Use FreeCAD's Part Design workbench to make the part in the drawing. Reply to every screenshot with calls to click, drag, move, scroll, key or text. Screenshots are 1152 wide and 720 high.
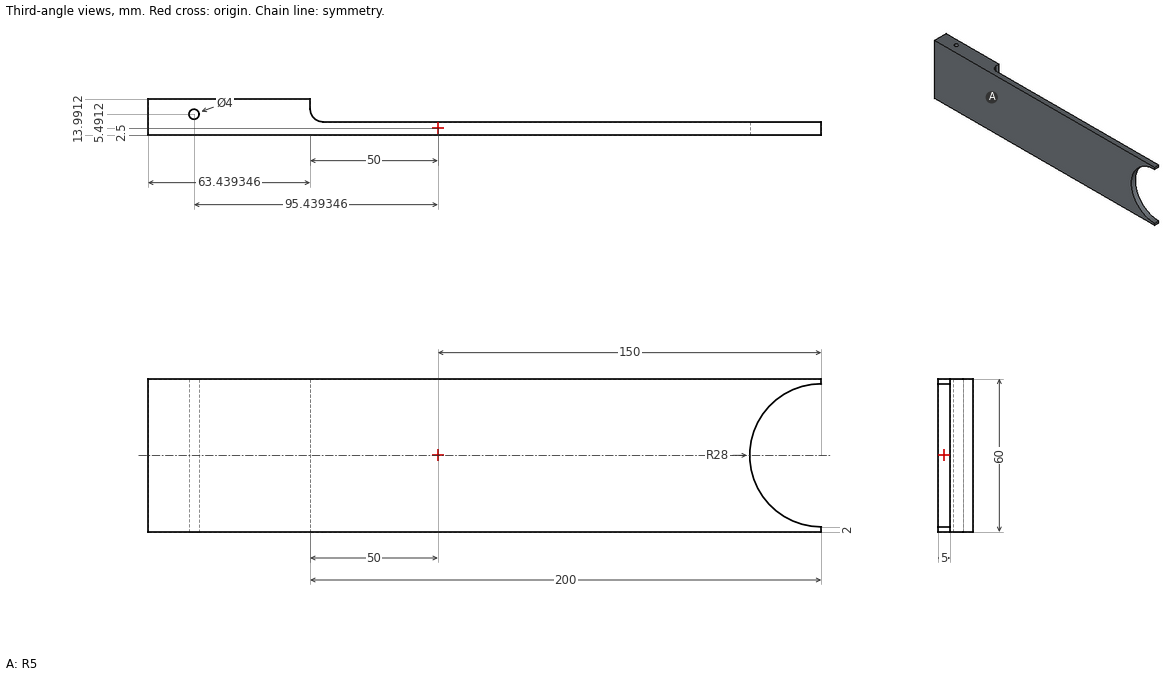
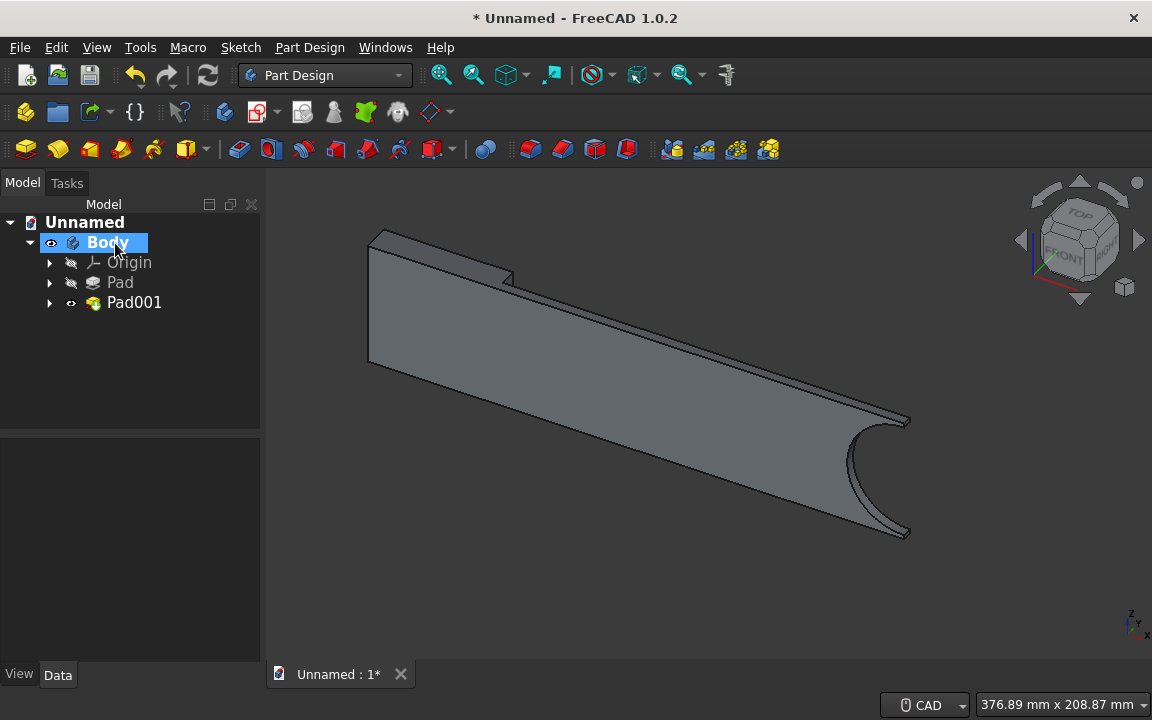
key(0)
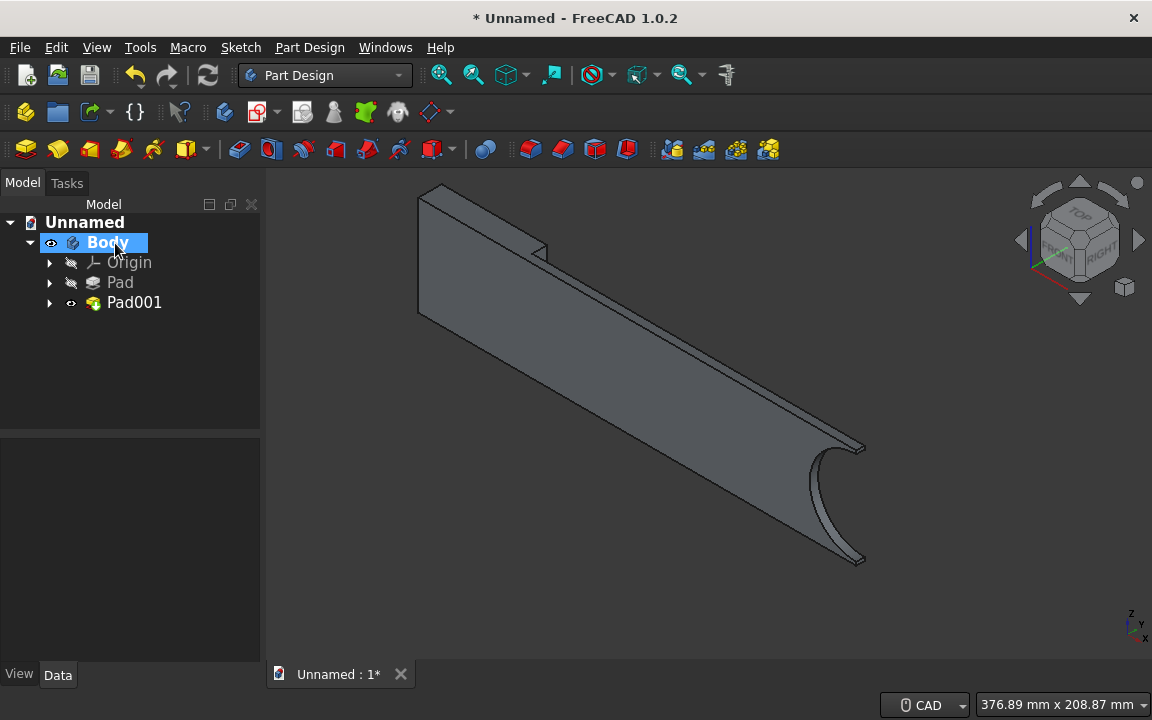
key(2)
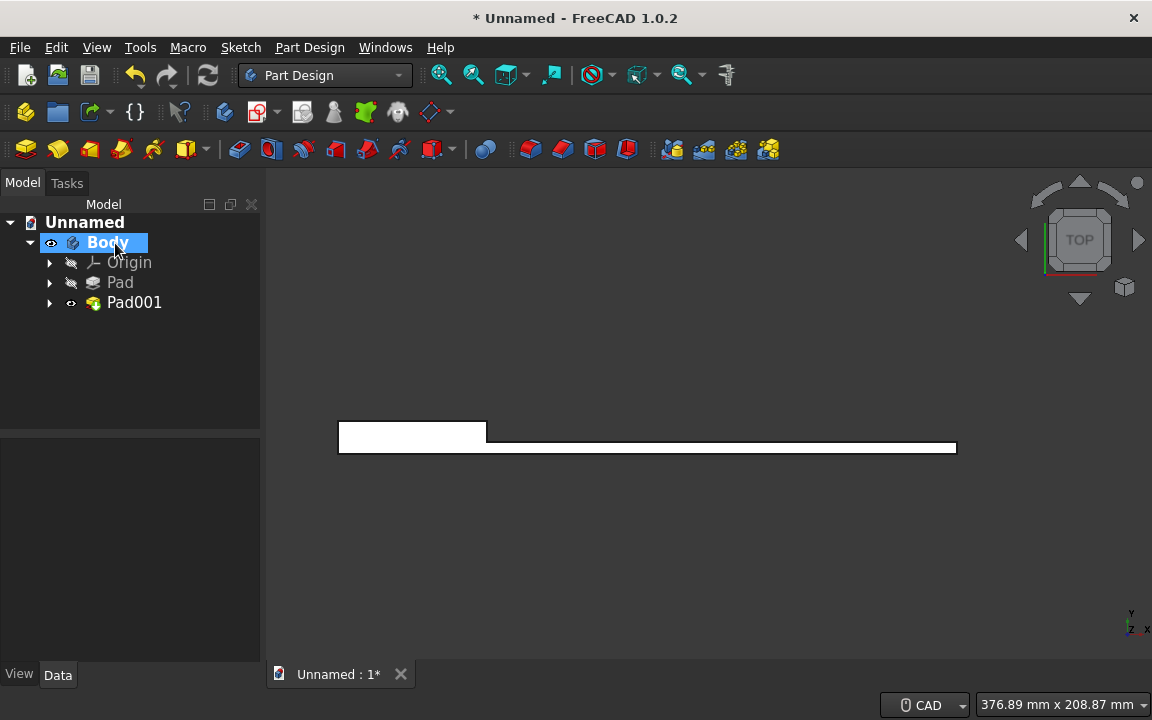
key(1)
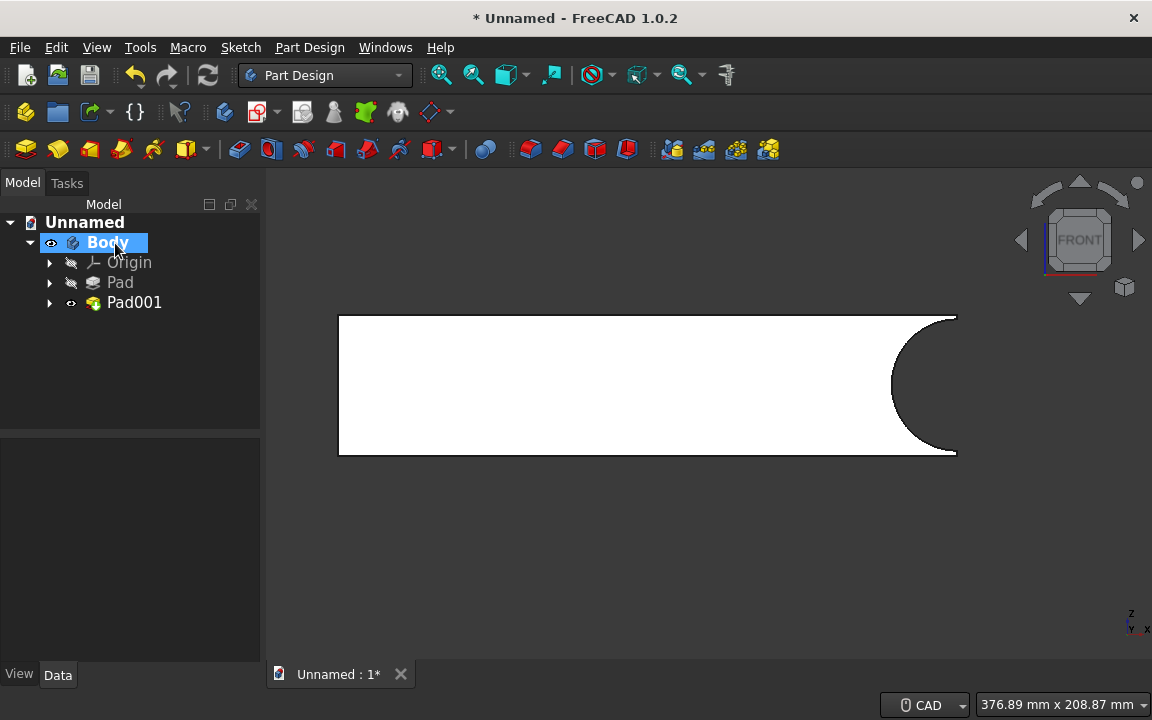
key(3)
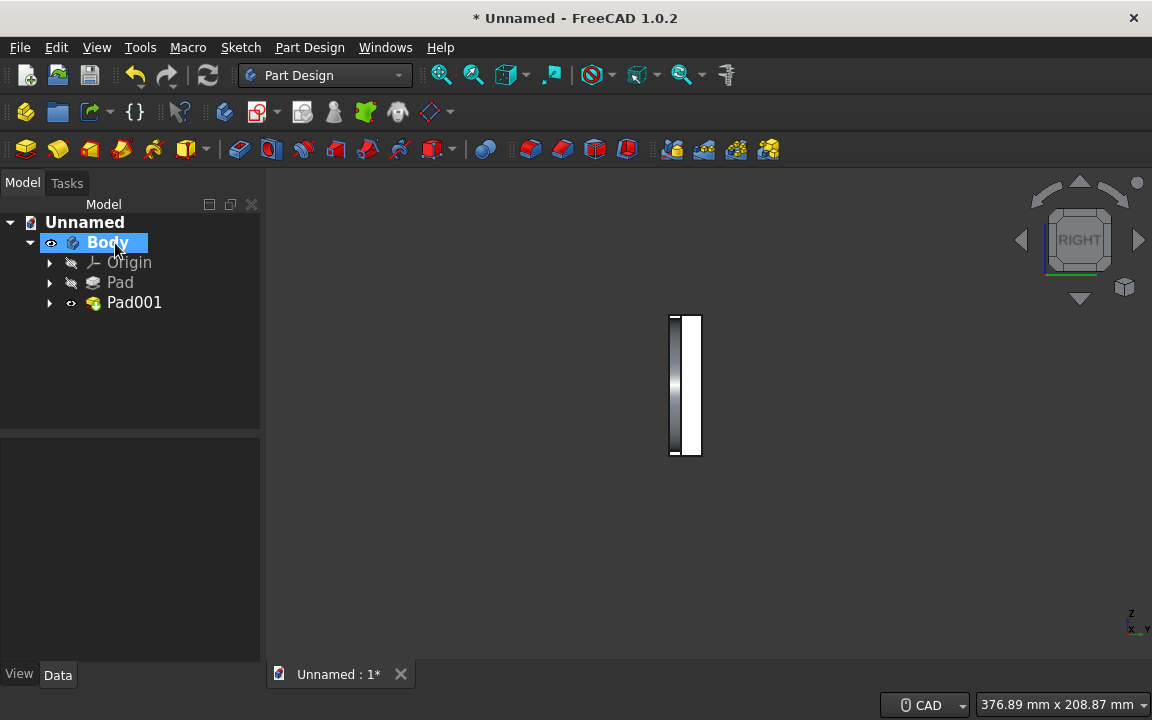
key(v)
key(f)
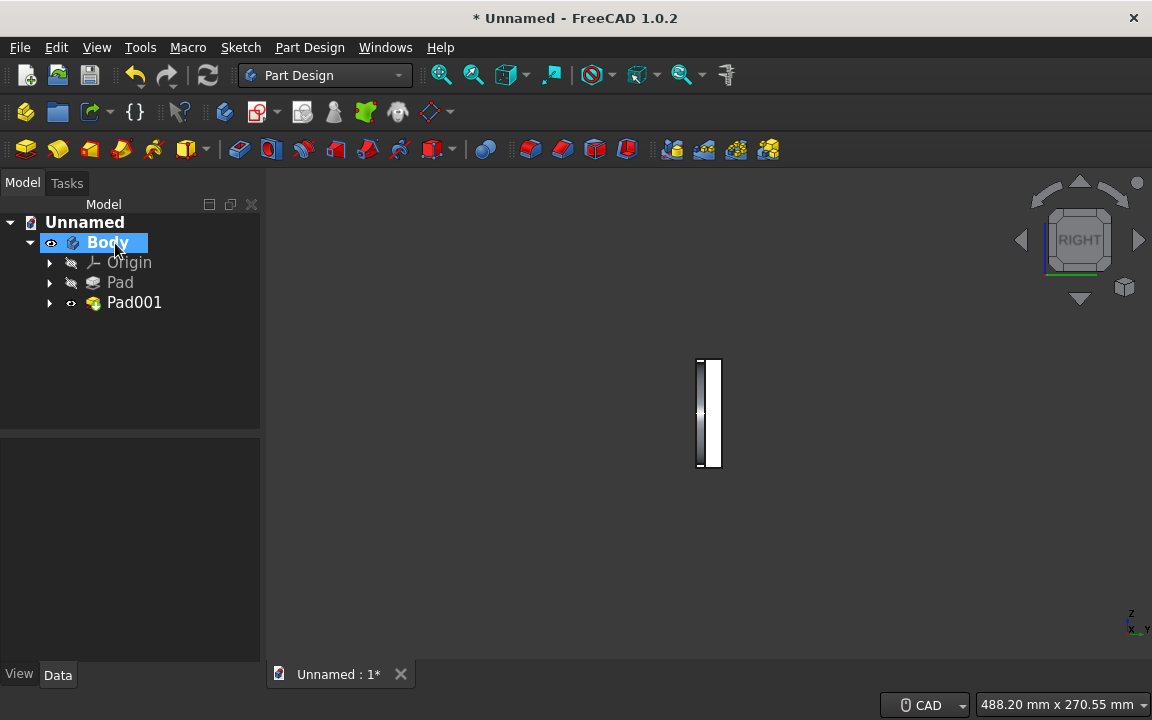
key(5)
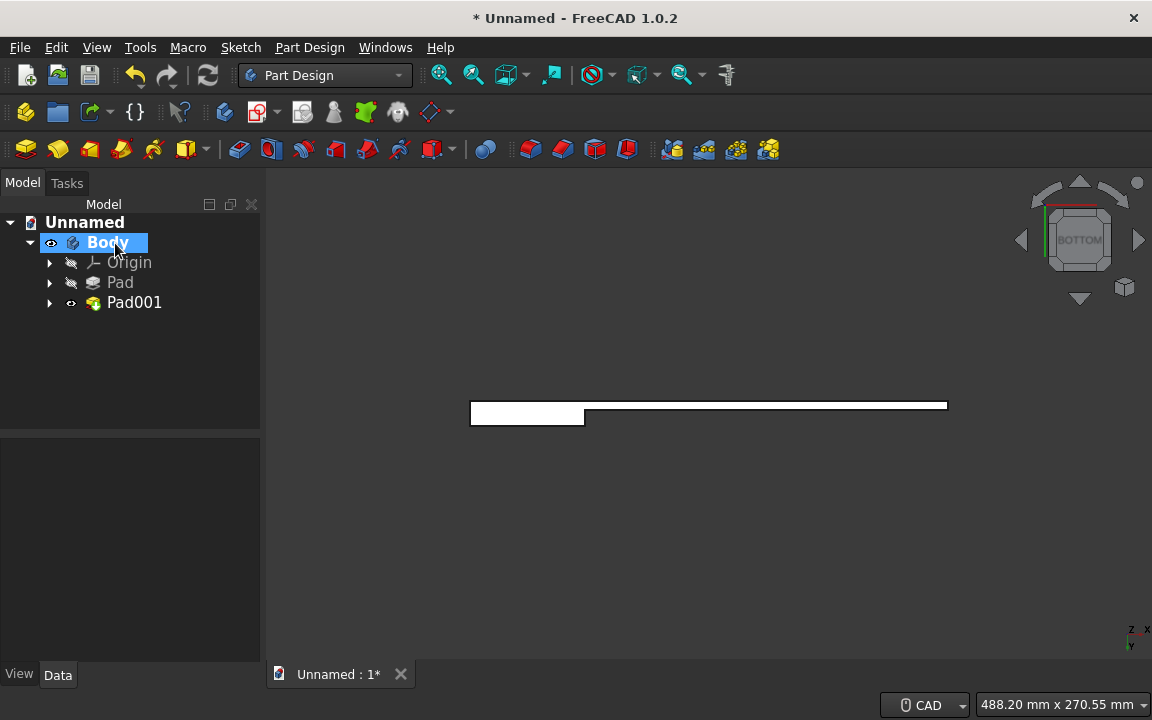
key(4)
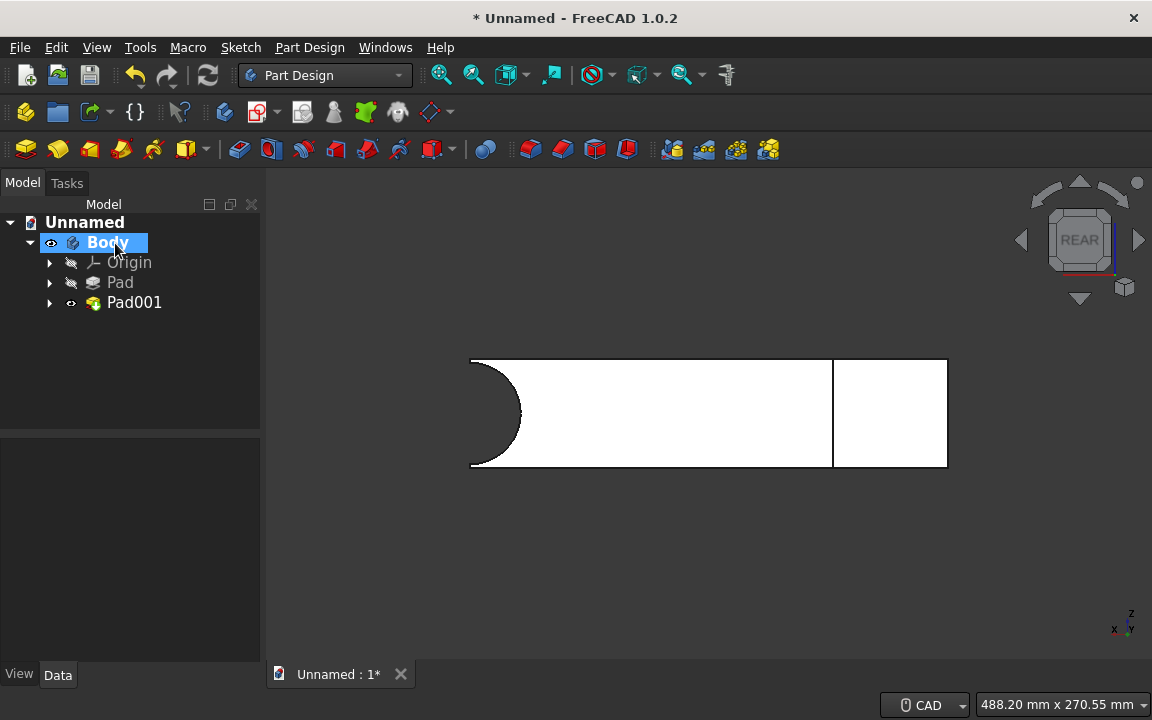
key(6)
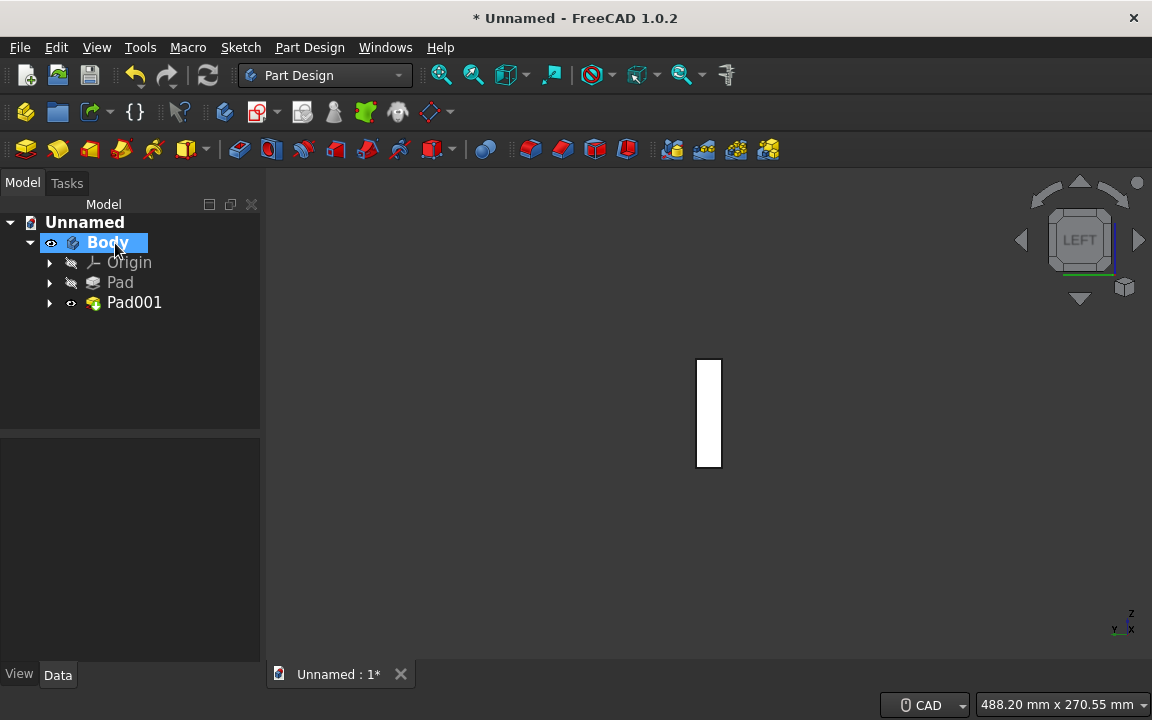
key(v)
key(f)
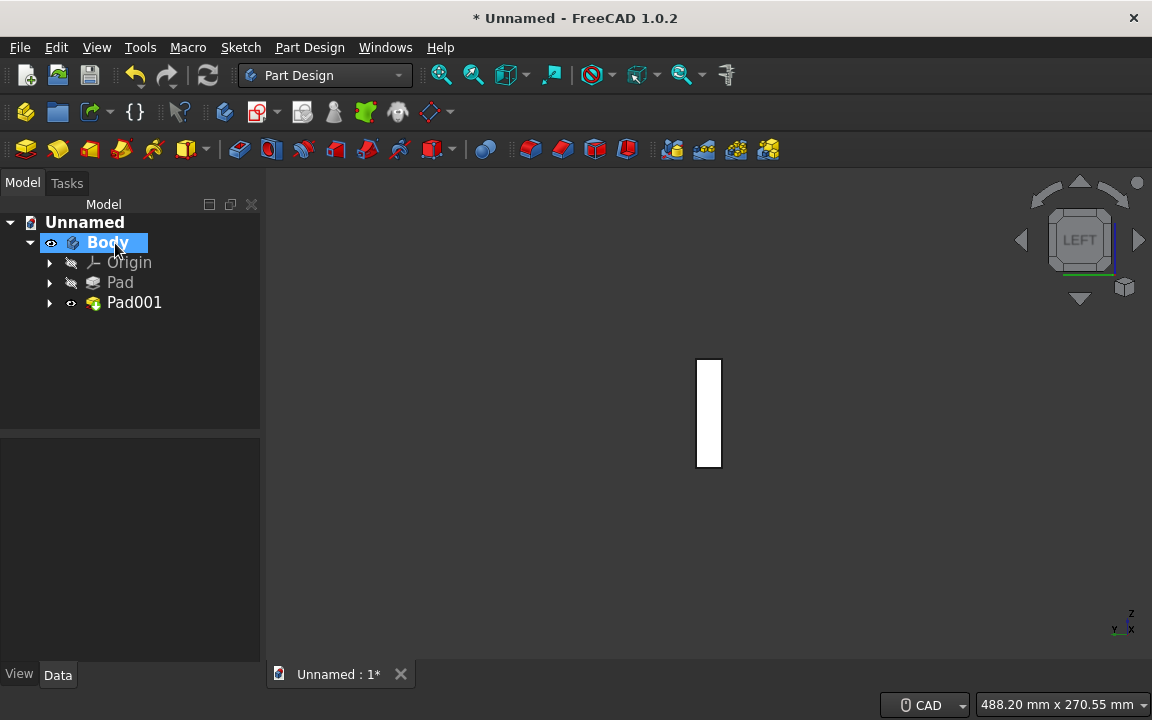
key(v)
key(3)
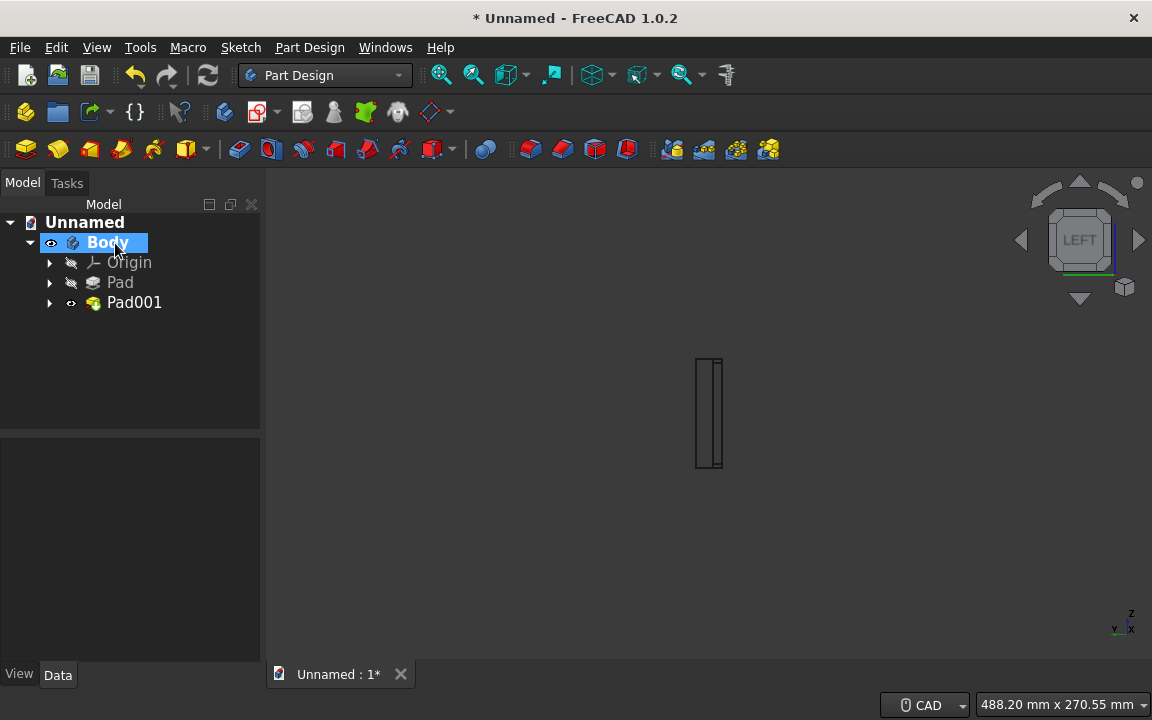
key(0)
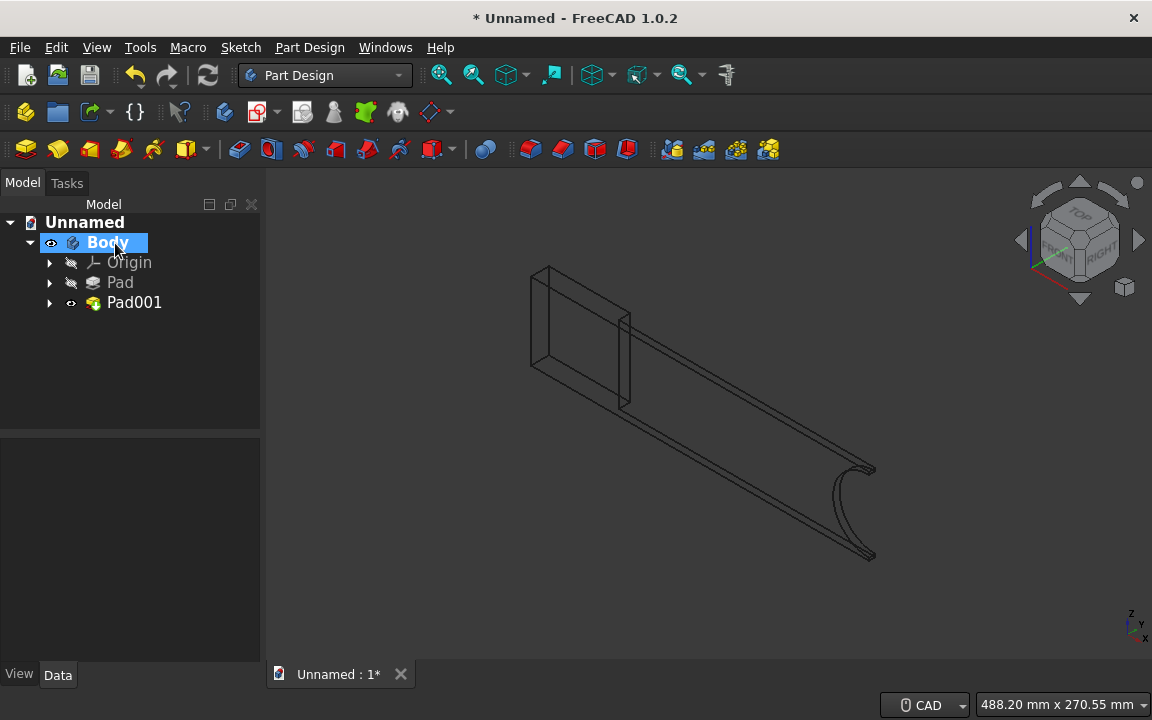
click(619, 363)